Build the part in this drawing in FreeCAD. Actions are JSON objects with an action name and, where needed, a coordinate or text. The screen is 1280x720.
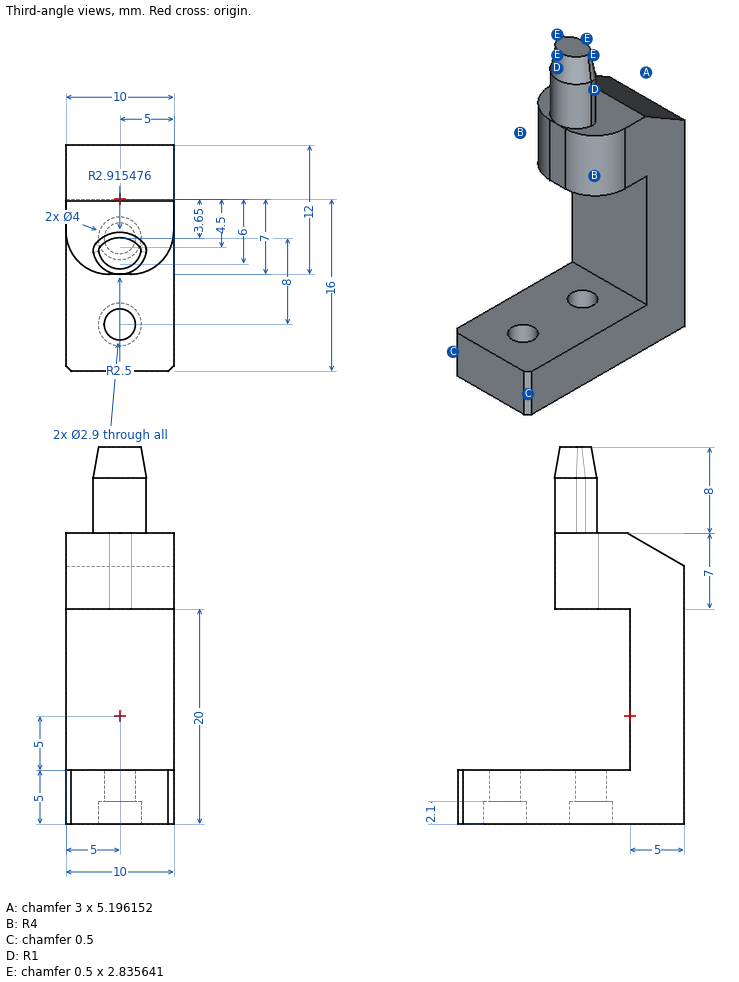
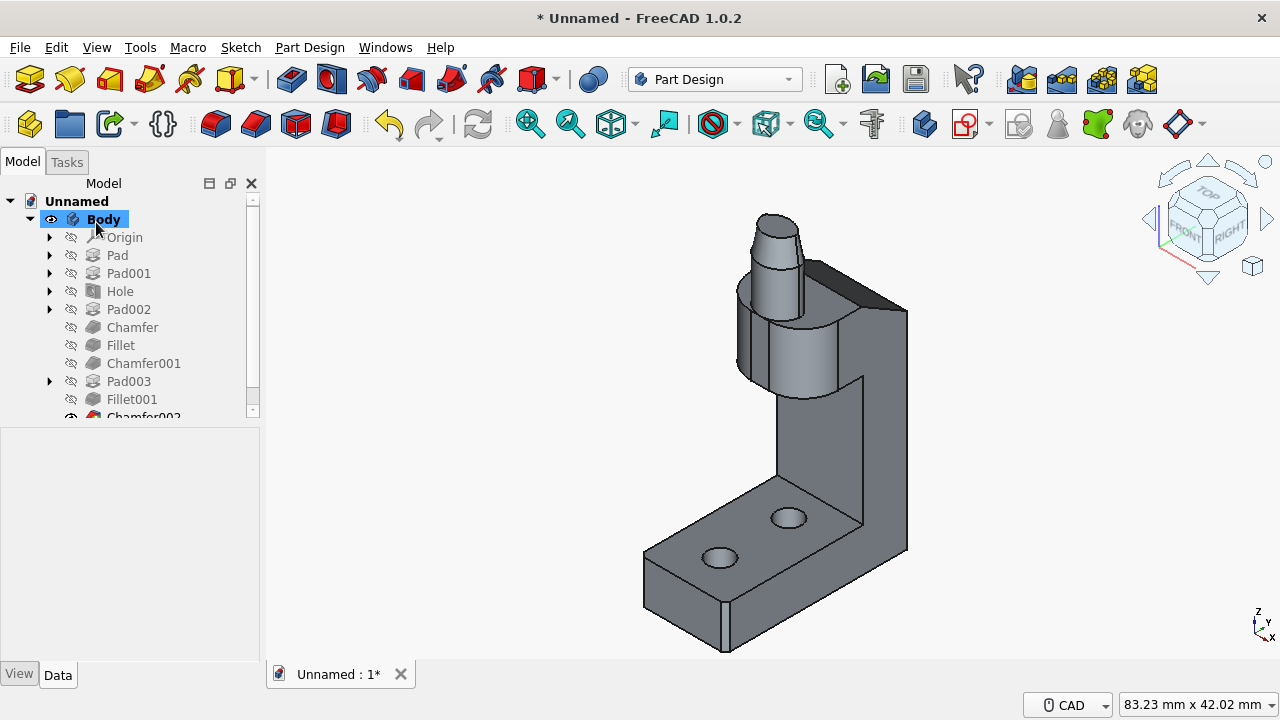
{"action": "key", "text": "5"}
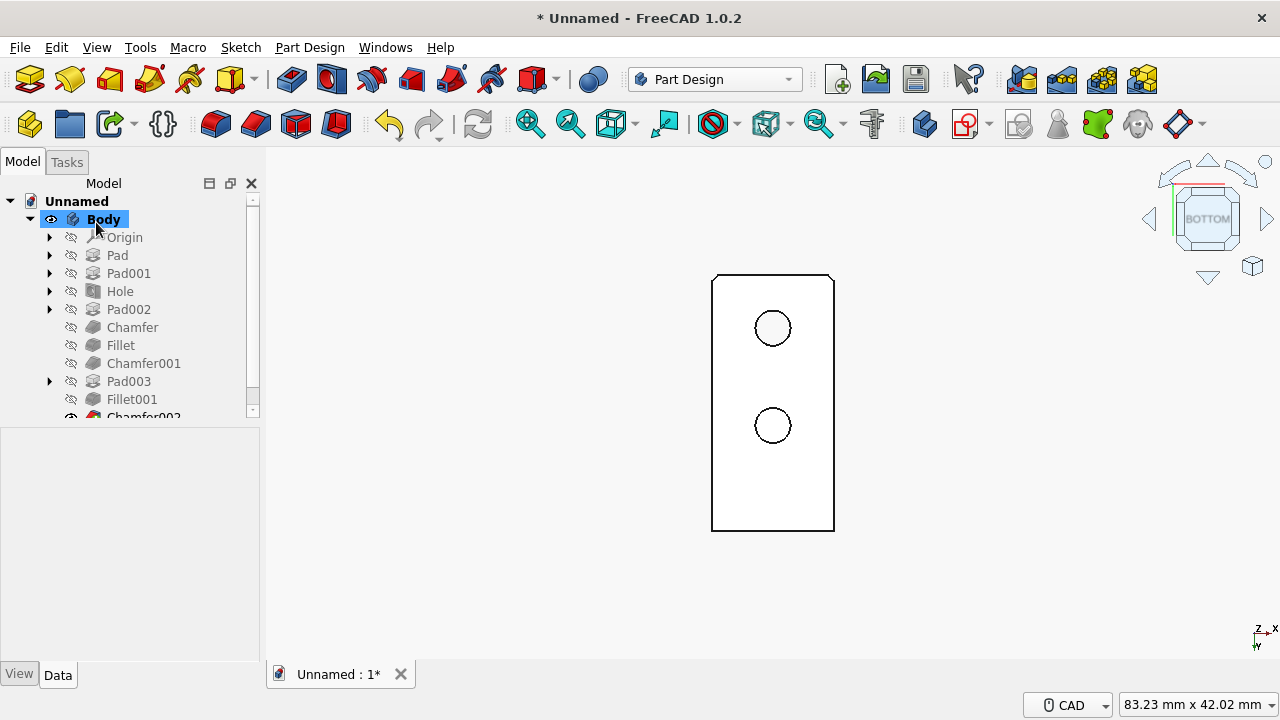
{"action": "left_click", "coordinate": [790, 475]}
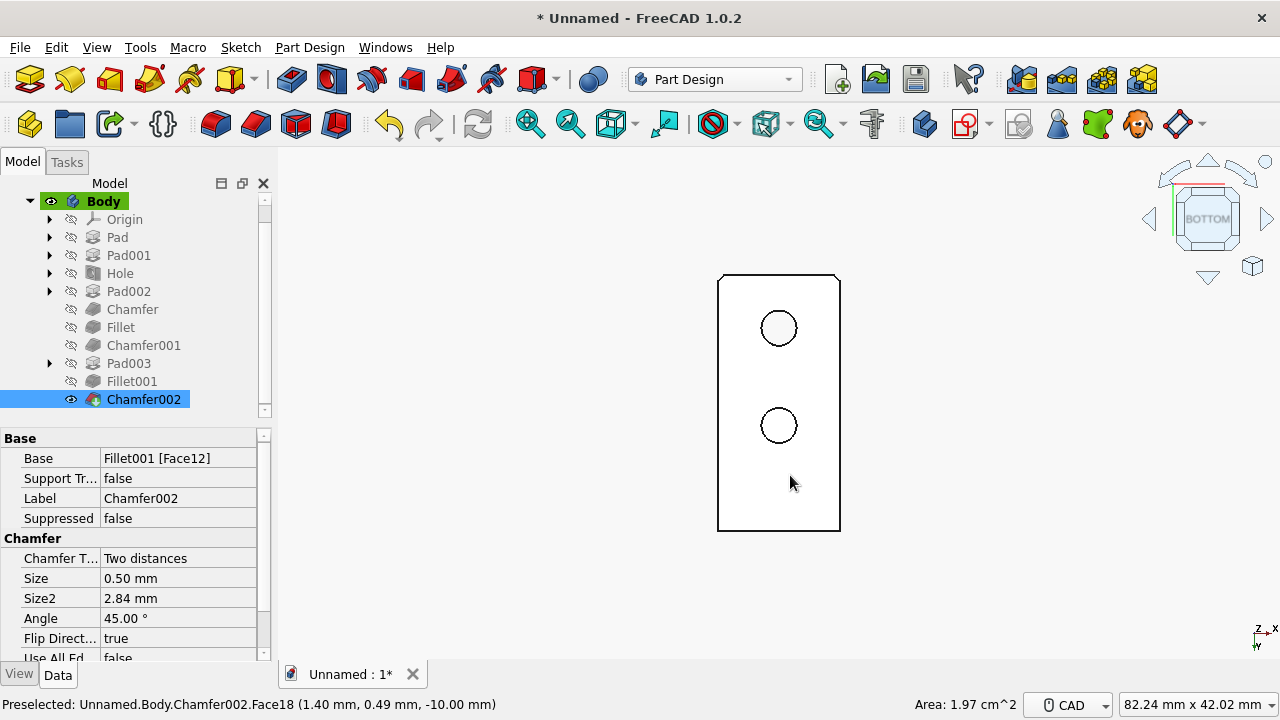
{"action": "left_click", "coordinate": [966, 124]}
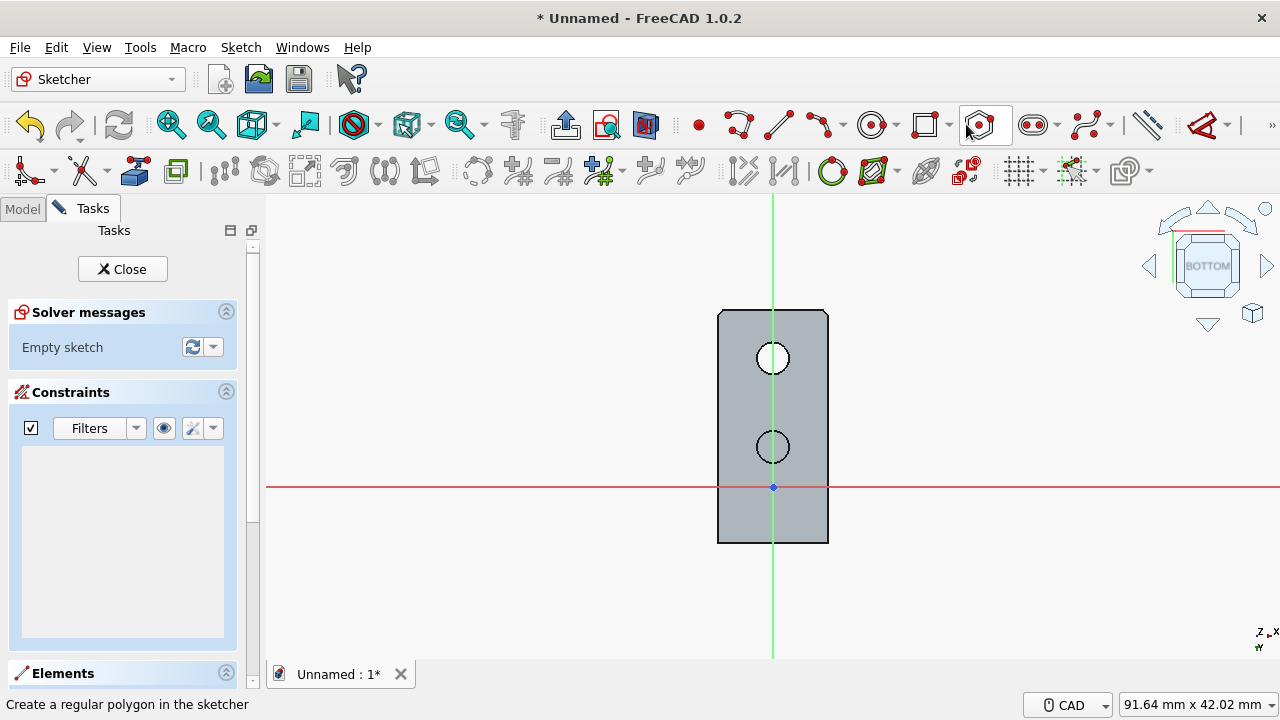
{"action": "scroll", "coordinate": [856, 394], "scroll_direction": "up", "scroll_amount": 3}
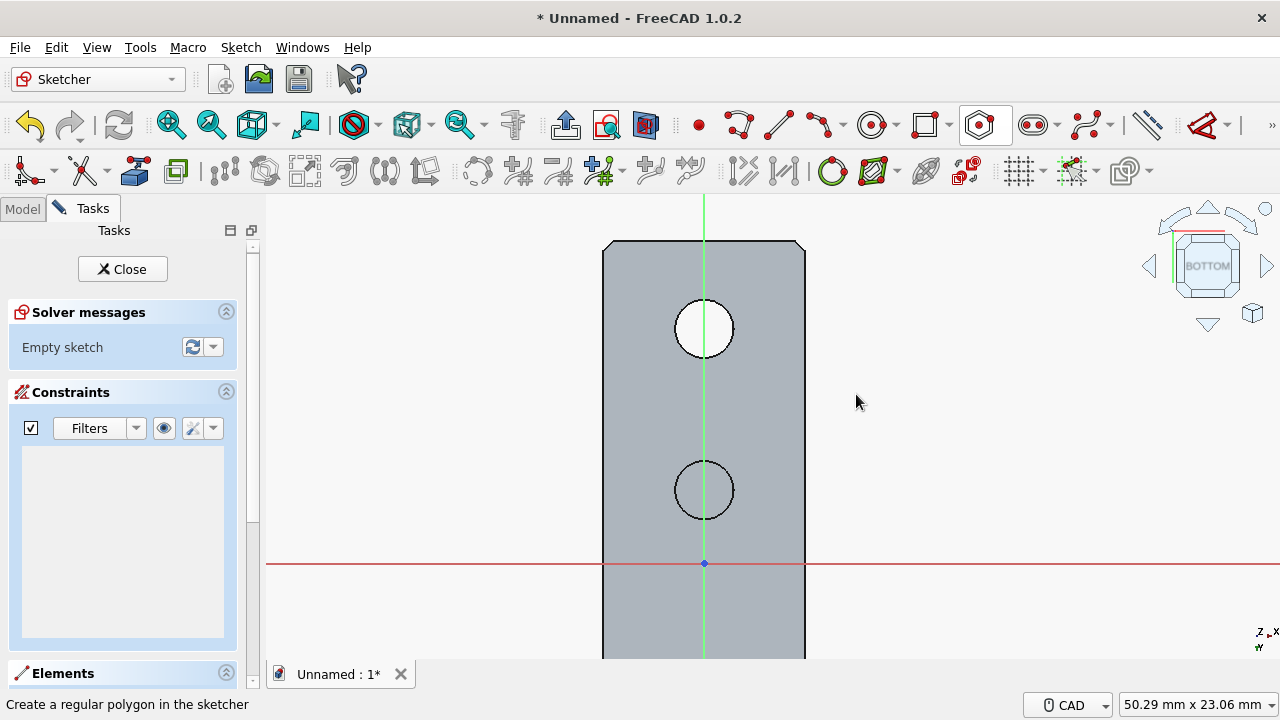
{"action": "key", "text": "g c"}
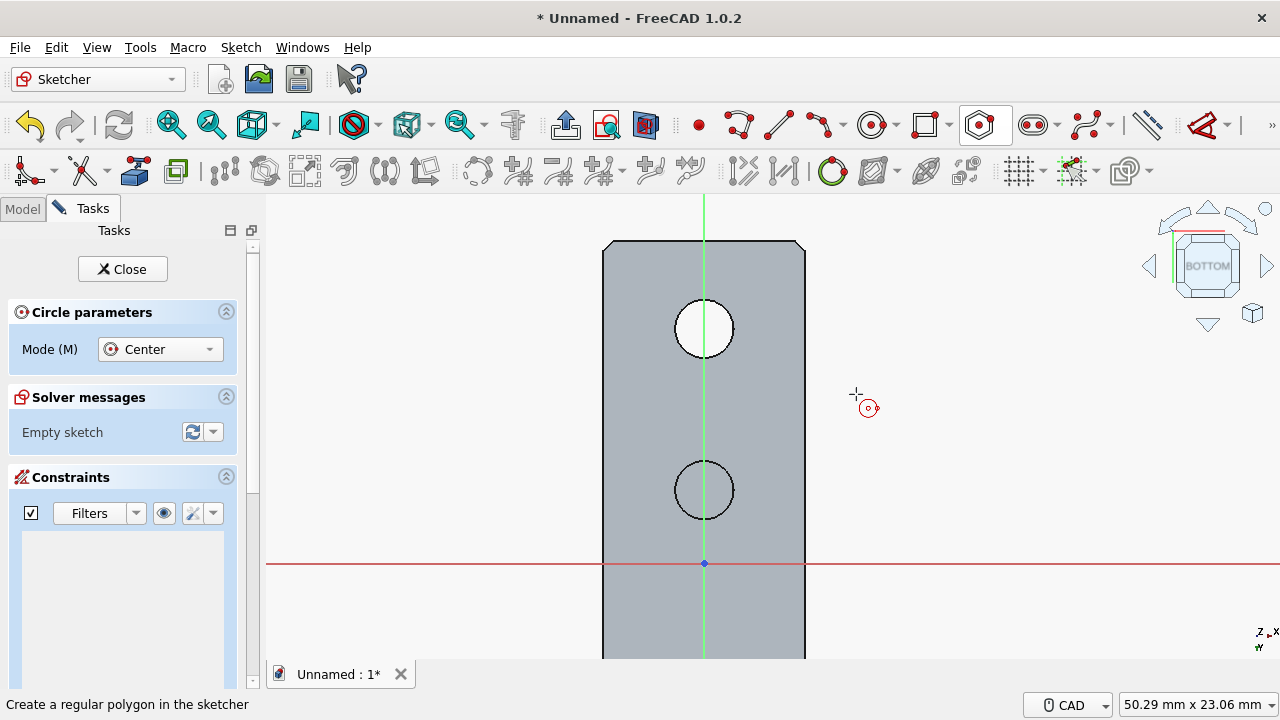
{"action": "left_click", "coordinate": [704, 490]}
{"action": "left_click", "coordinate": [733, 462]}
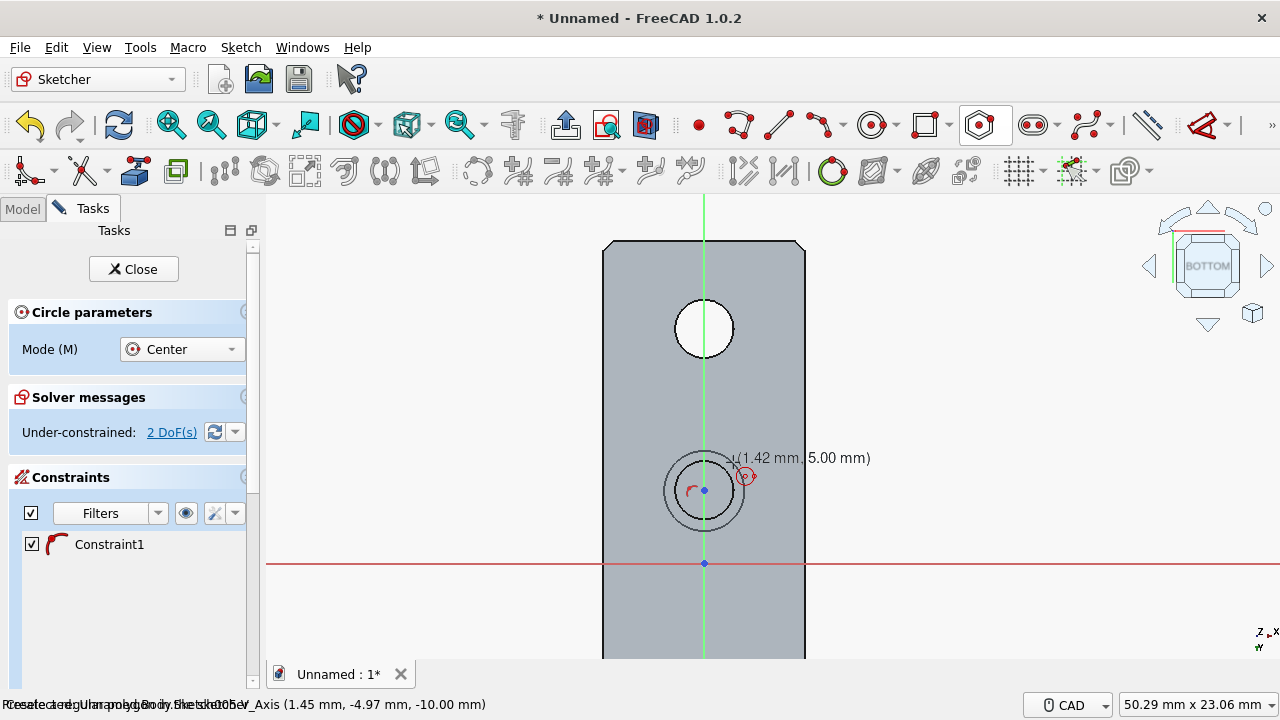
{"action": "left_click", "coordinate": [704, 329]}
{"action": "left_click", "coordinate": [733, 300]}
{"action": "key", "text": "Escape"}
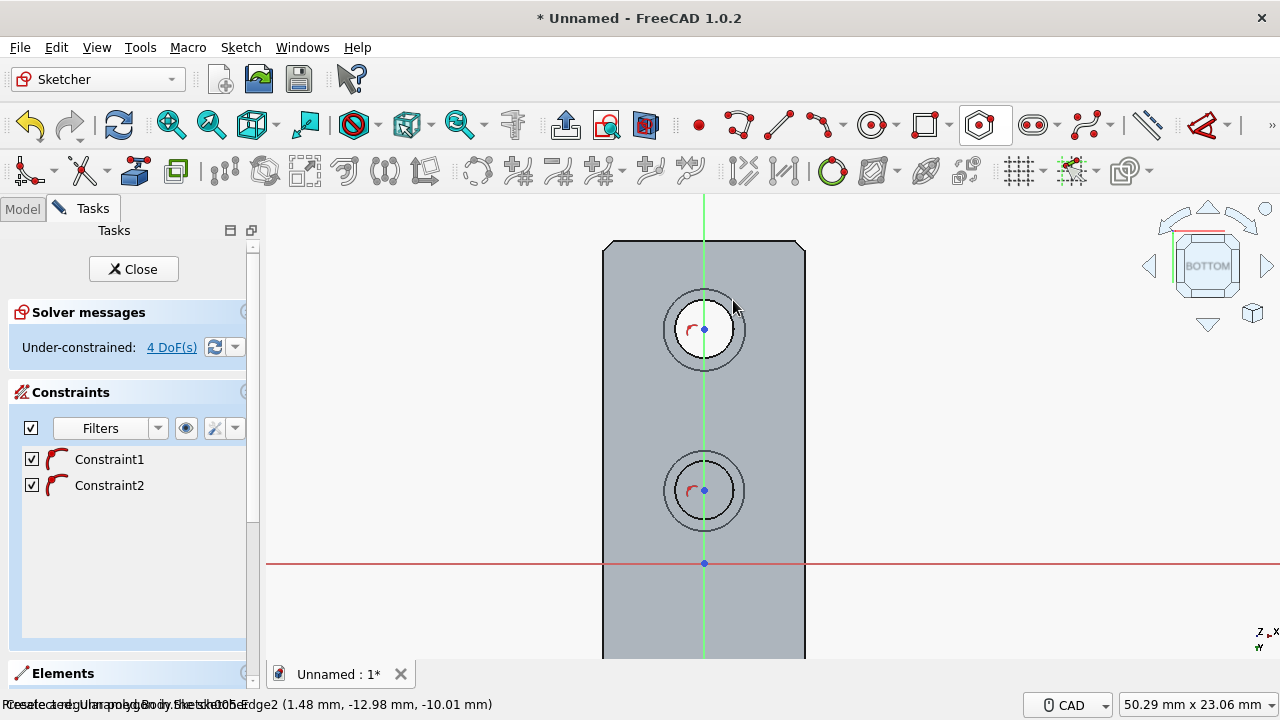
{"action": "left_click", "coordinate": [733, 463]}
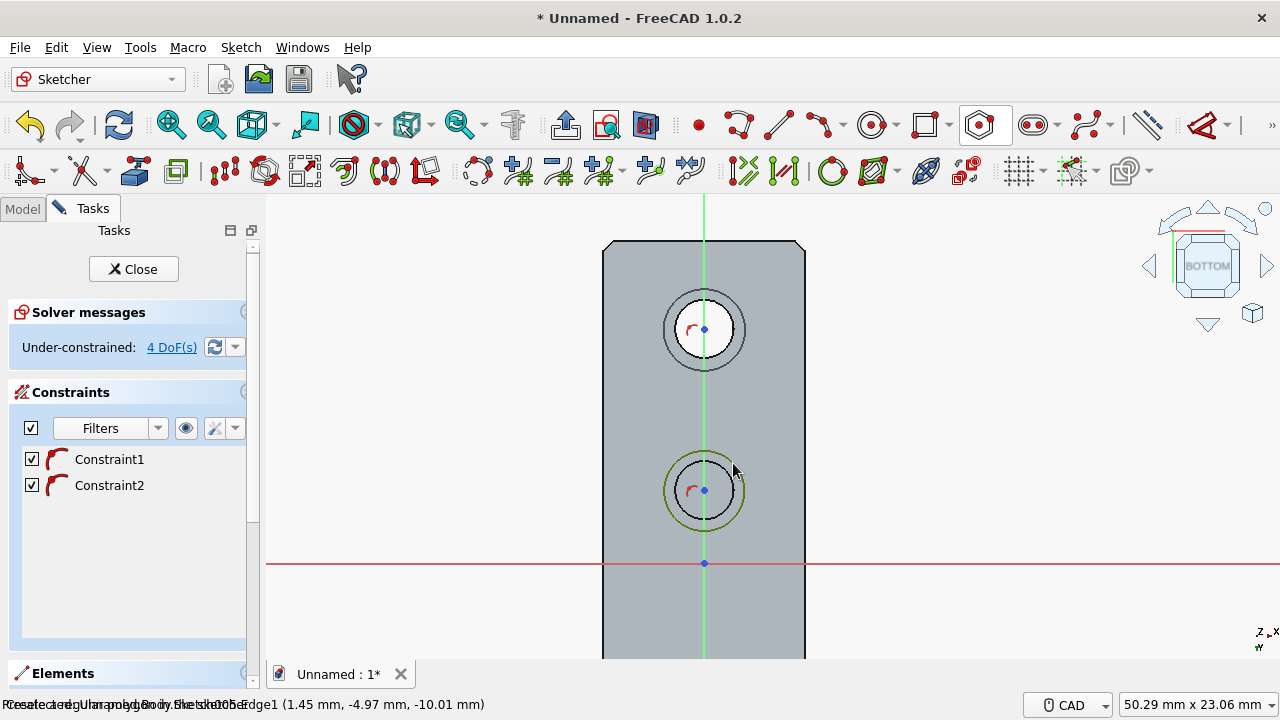
{"action": "left_click", "coordinate": [733, 301]}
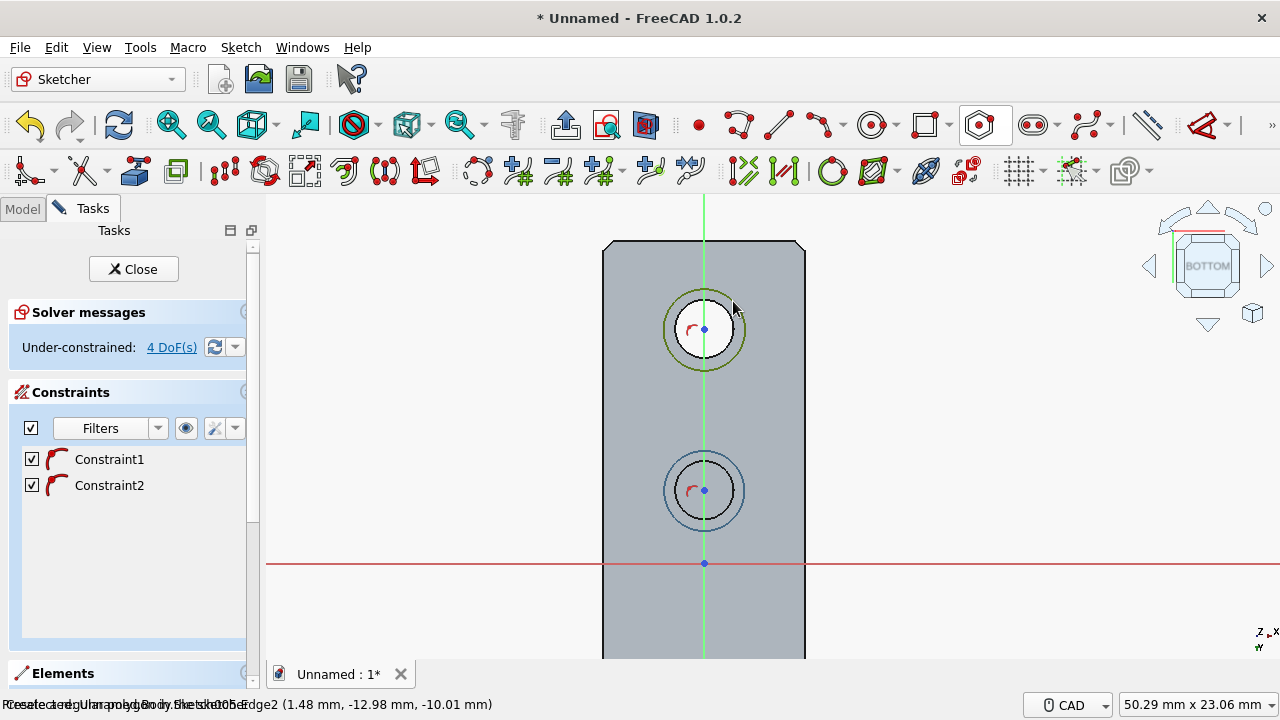
{"action": "key", "text": "e"}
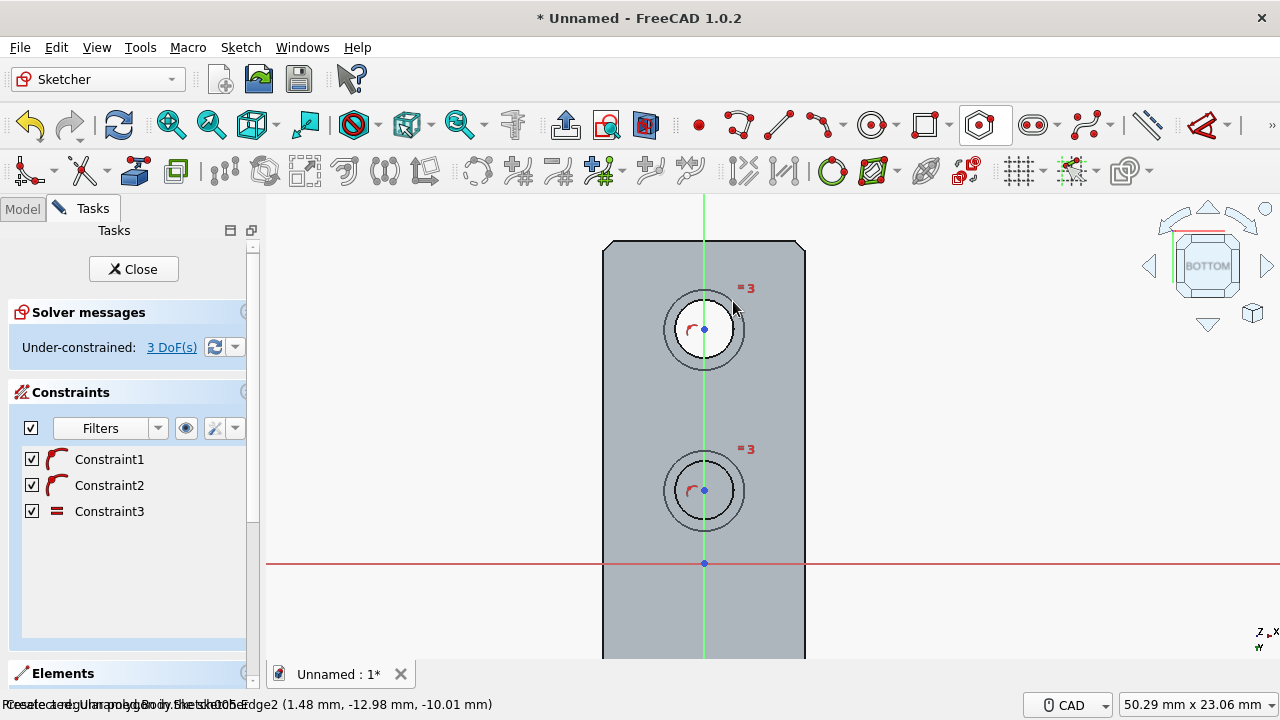
{"action": "left_click", "coordinate": [1202, 126]}